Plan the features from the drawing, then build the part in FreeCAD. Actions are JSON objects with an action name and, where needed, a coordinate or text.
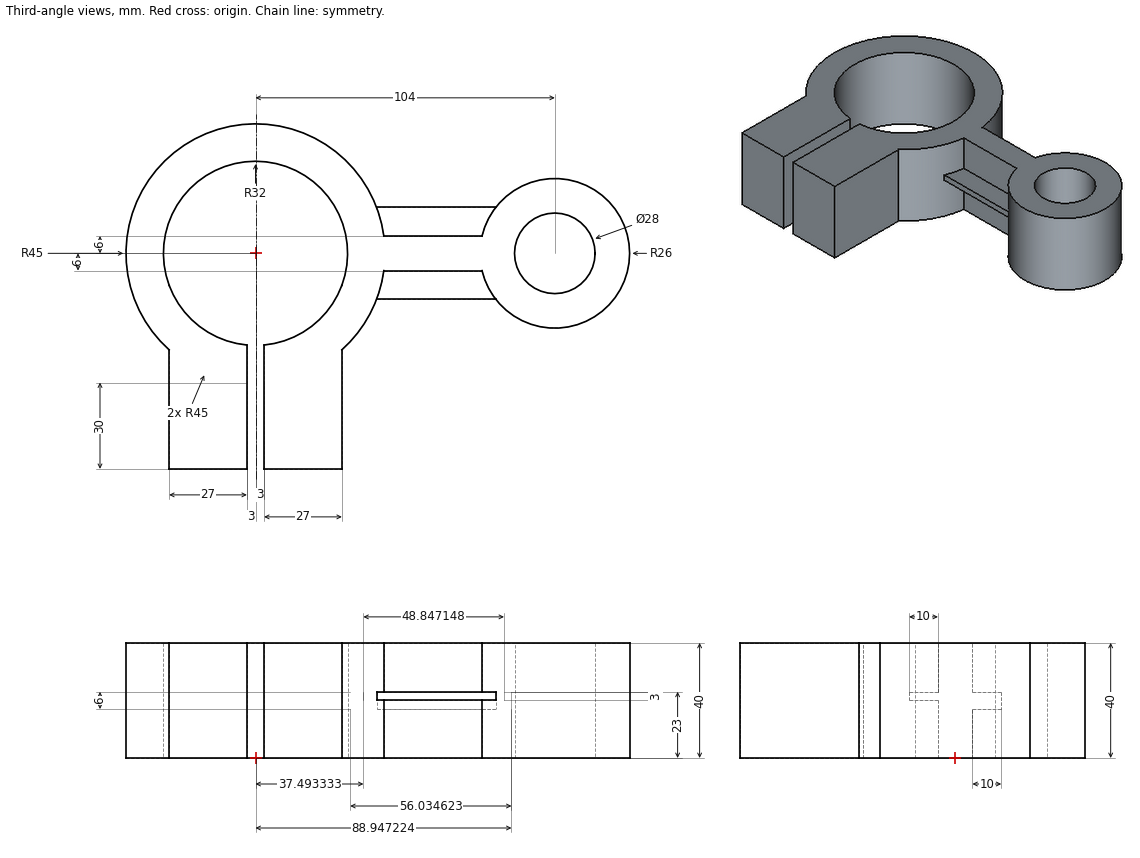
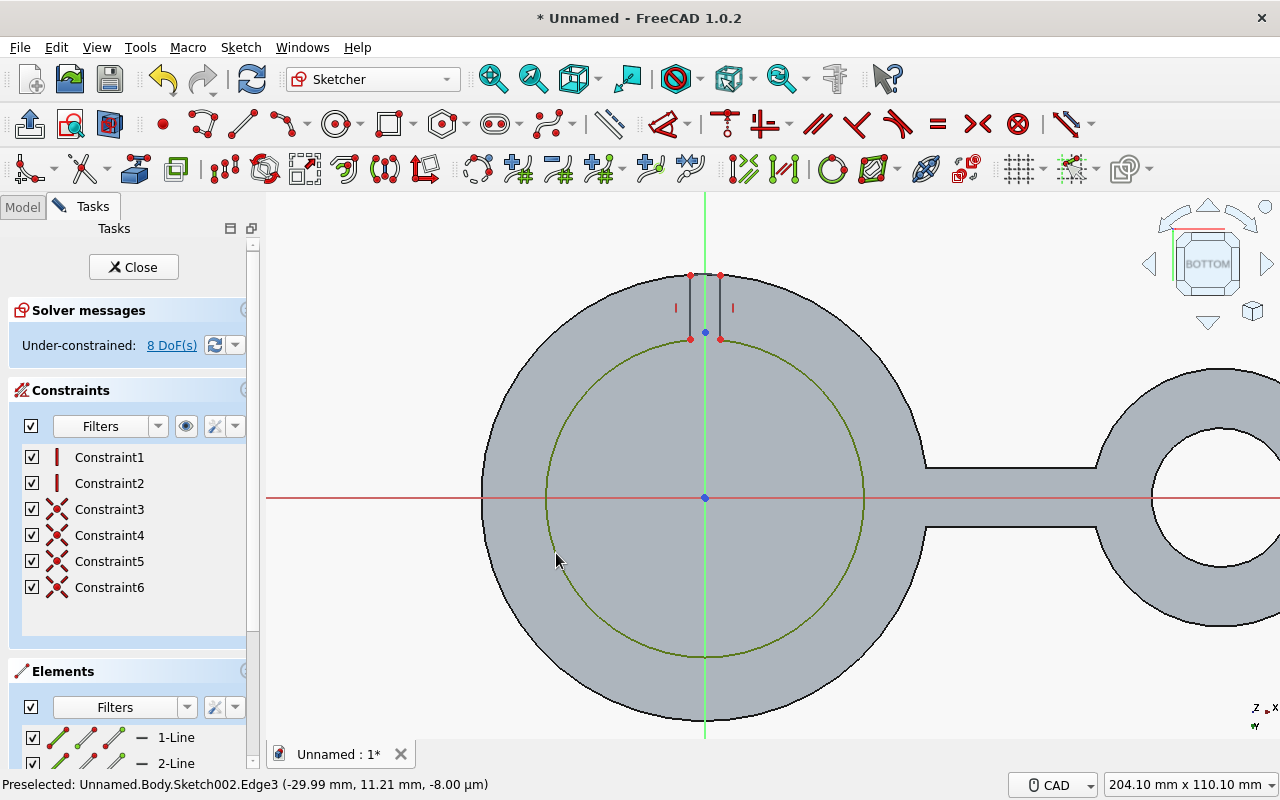
{"action": "left_click", "coordinate": [705, 274]}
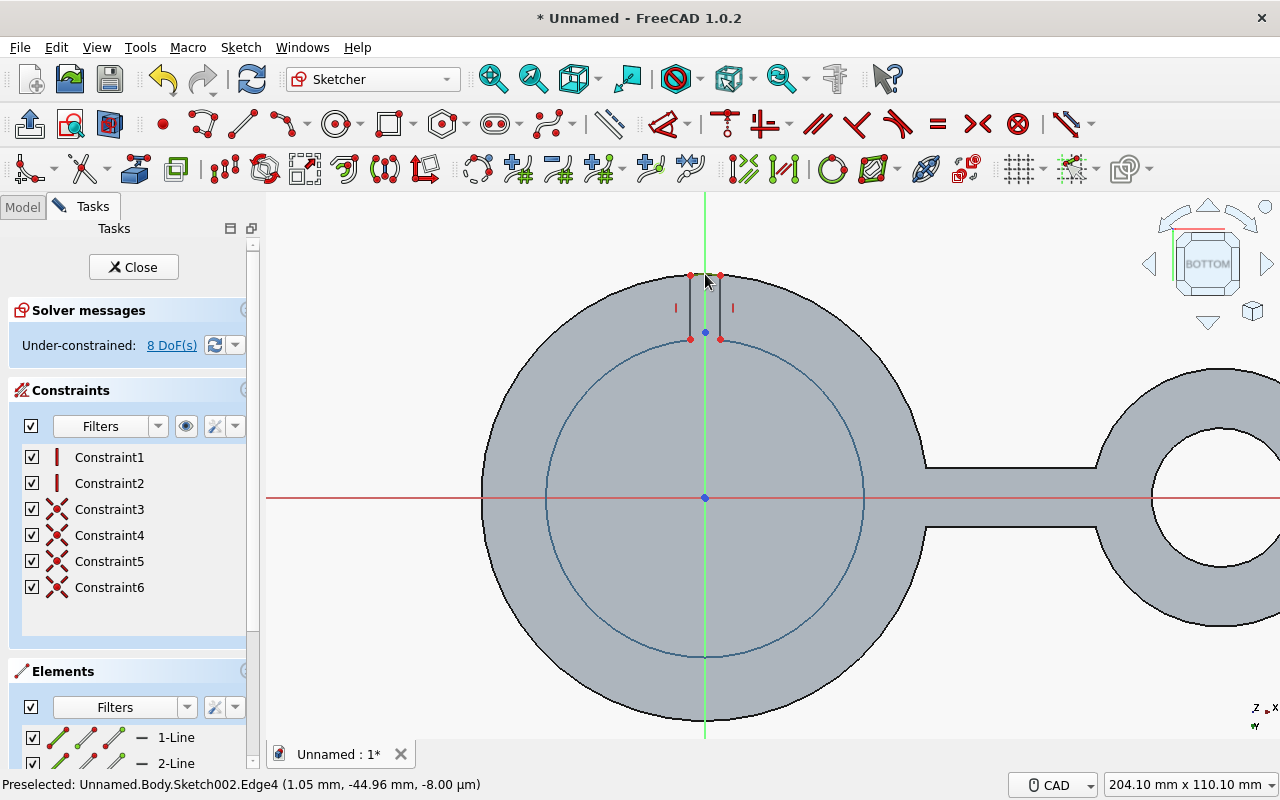
{"action": "key", "text": "c"}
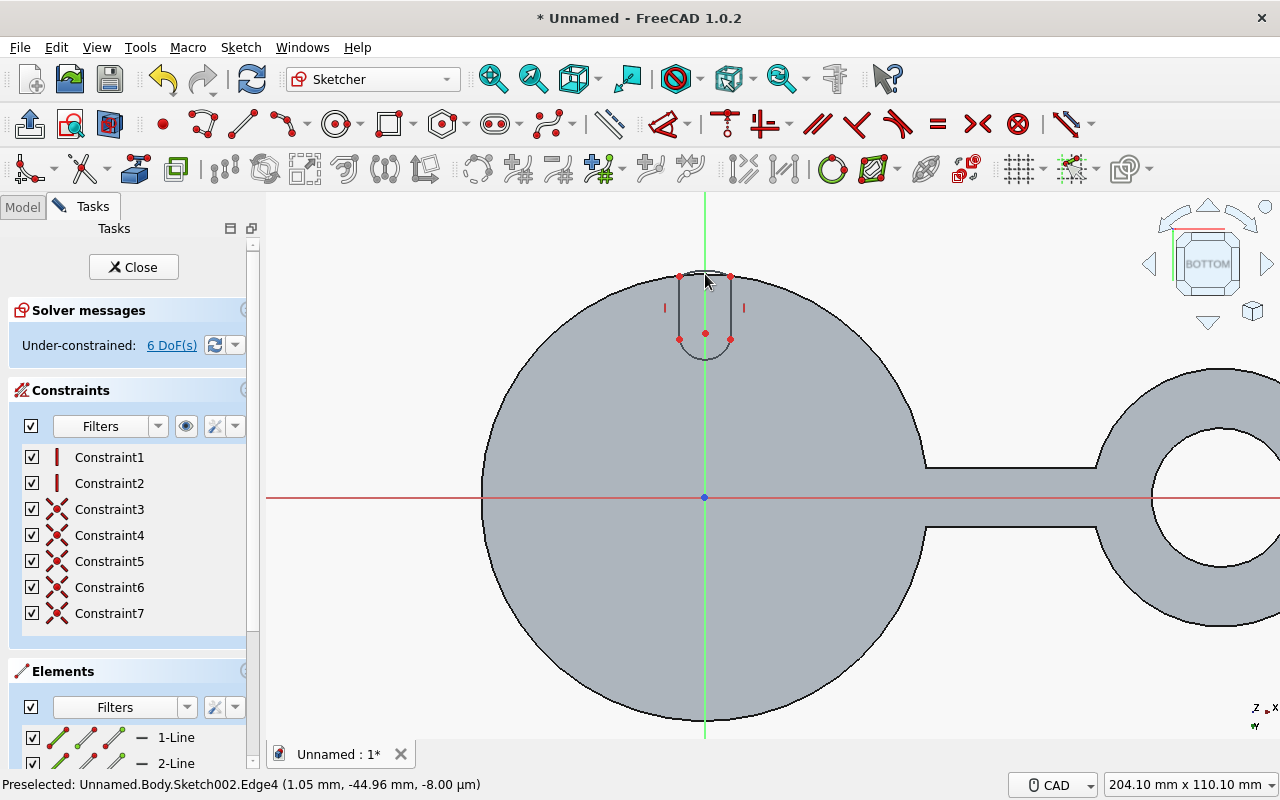
{"action": "scroll", "coordinate": [705, 415], "scroll_direction": "up", "scroll_amount": 3}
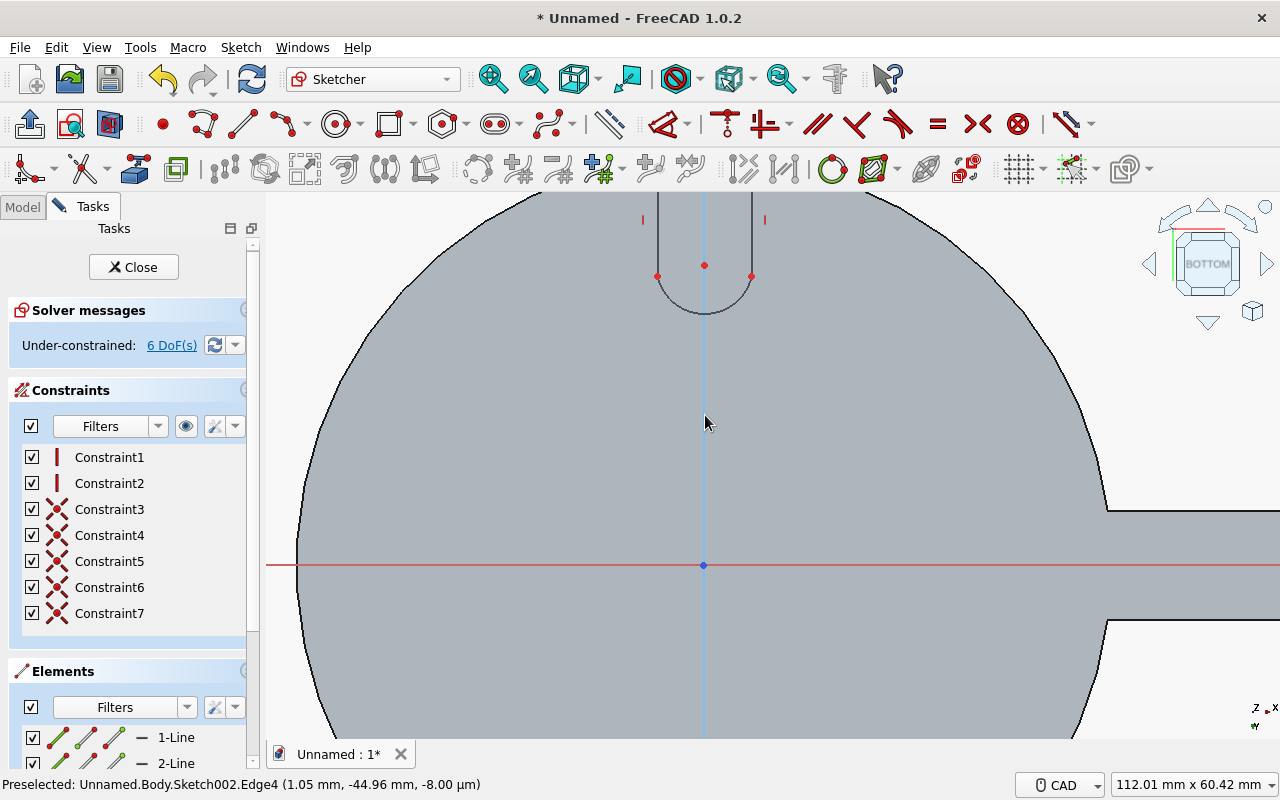
{"action": "left_click_drag", "start_coordinate": [694, 256], "coordinate": [715, 575]}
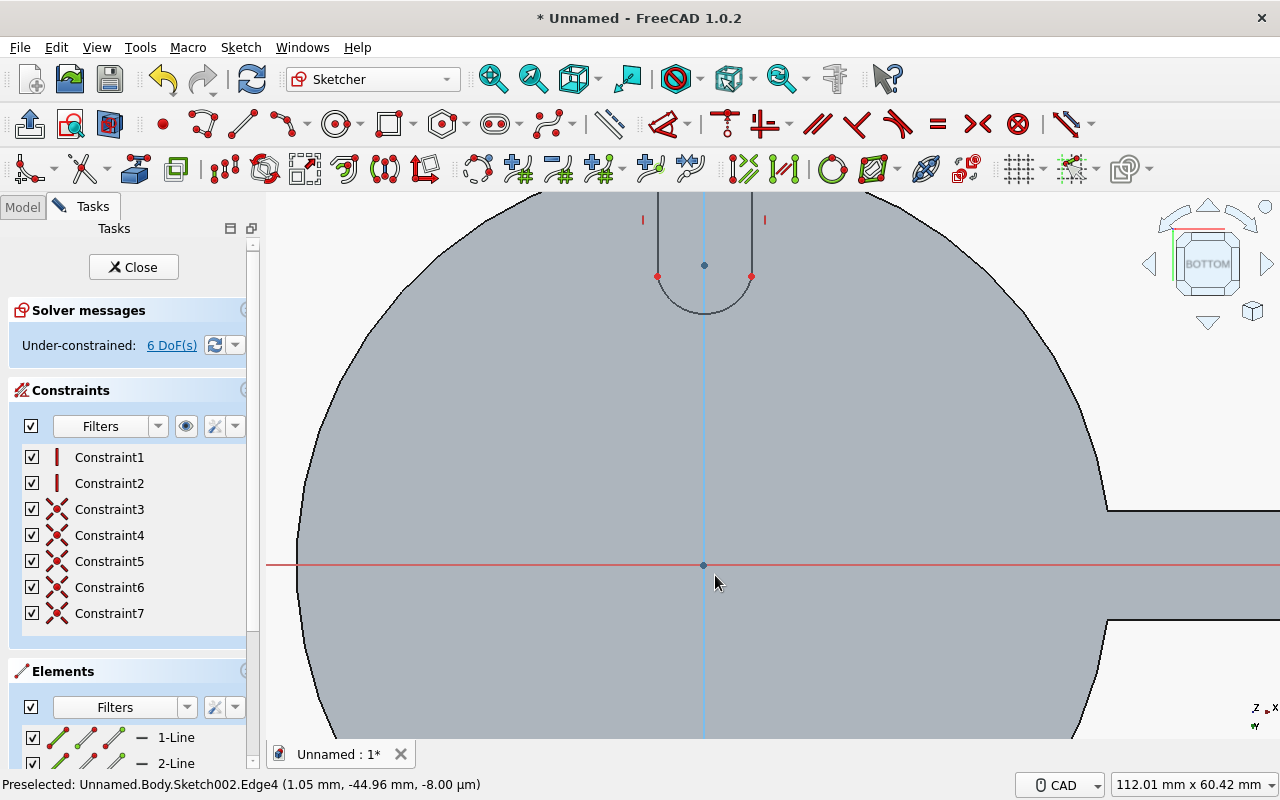
{"action": "left_click", "coordinate": [726, 124]}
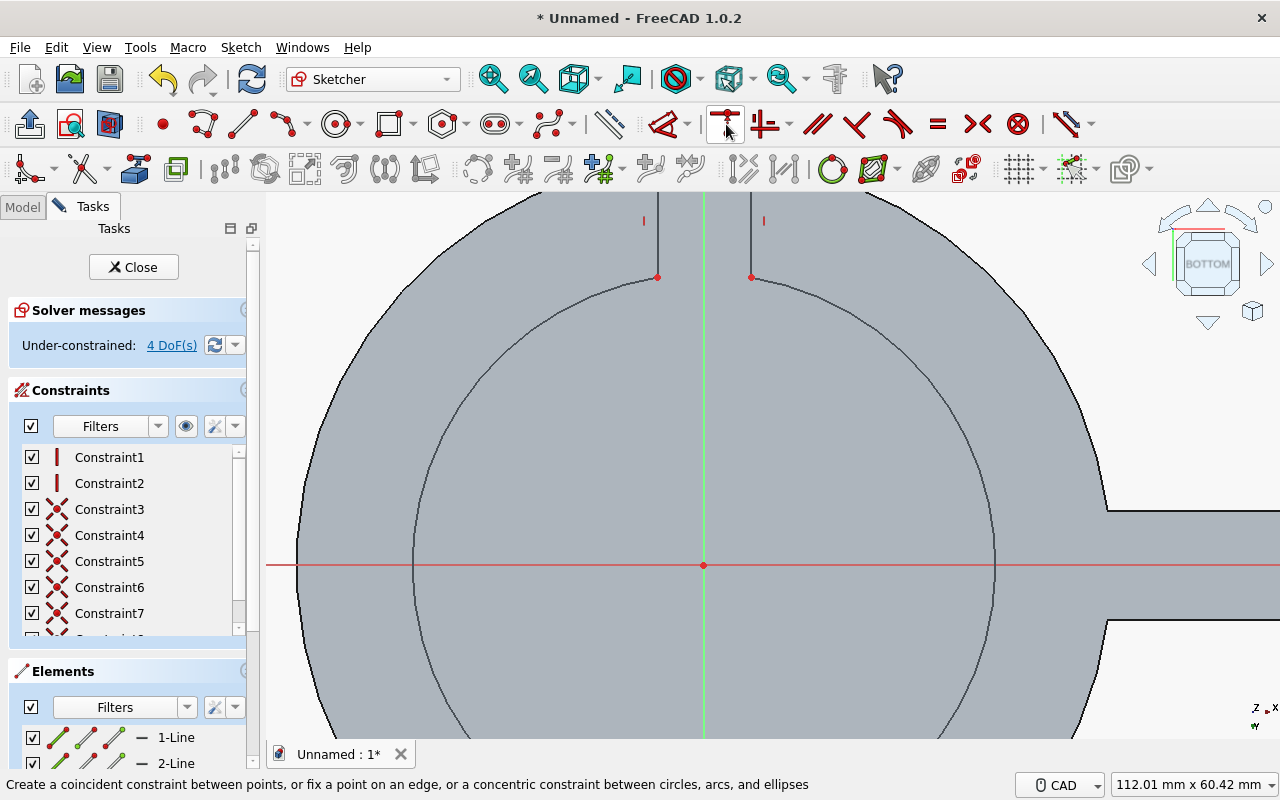
{"action": "key", "text": "d"}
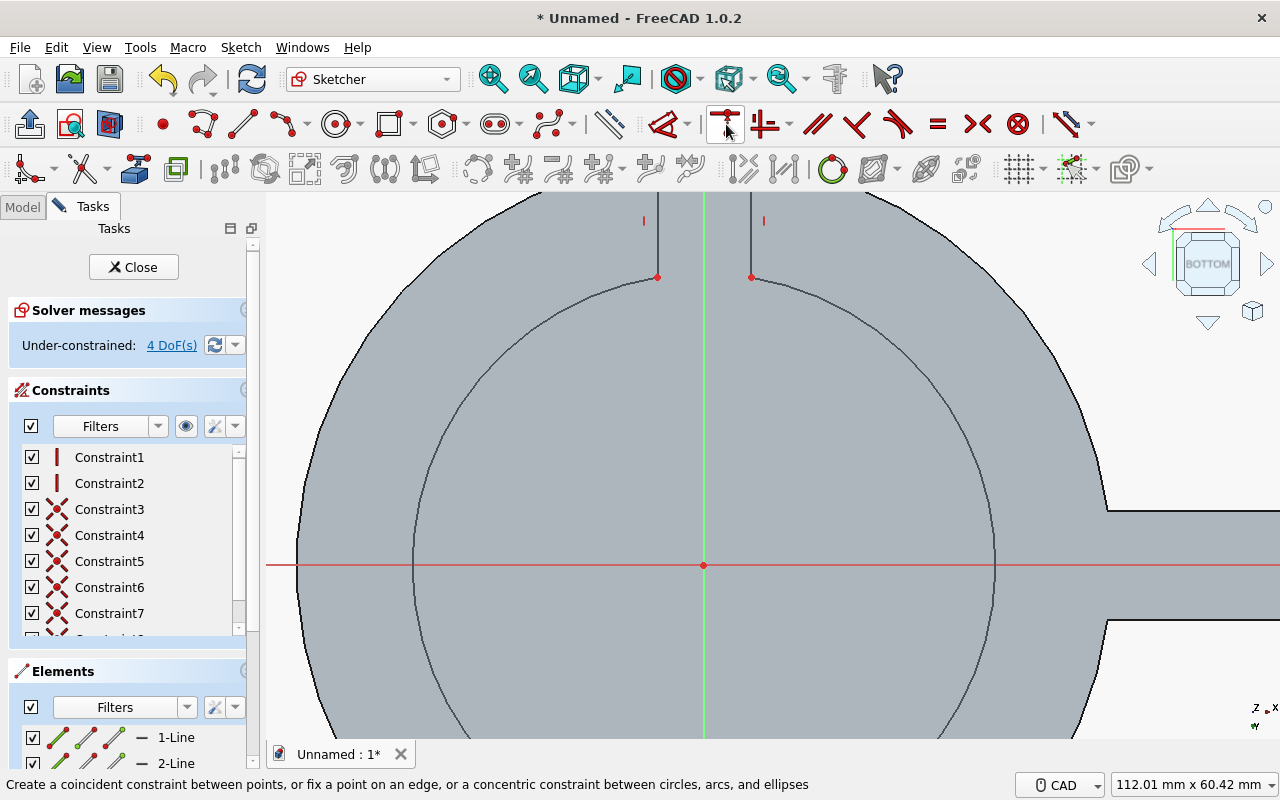
{"action": "left_click", "coordinate": [433, 672]}
{"action": "left_click", "coordinate": [403, 684]}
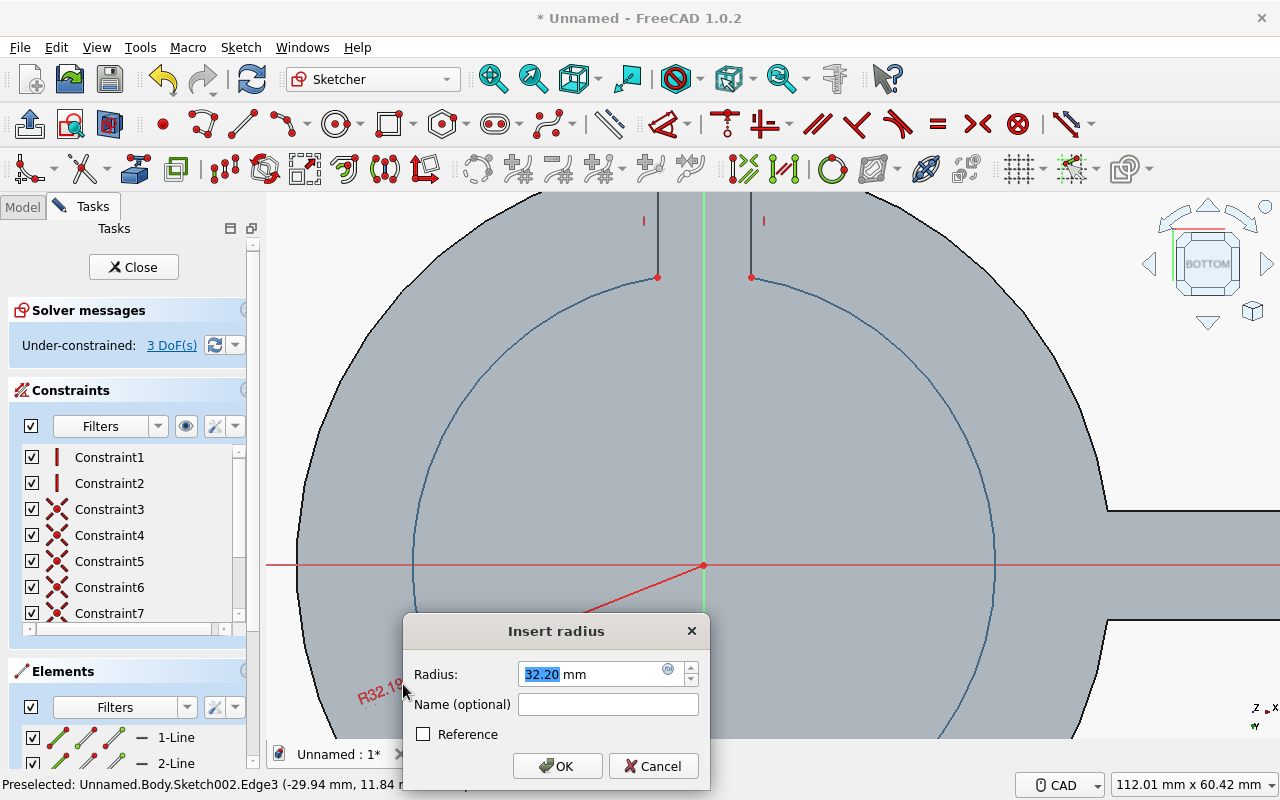
{"action": "type", "text": "32"}
{"action": "key", "text": "Return"}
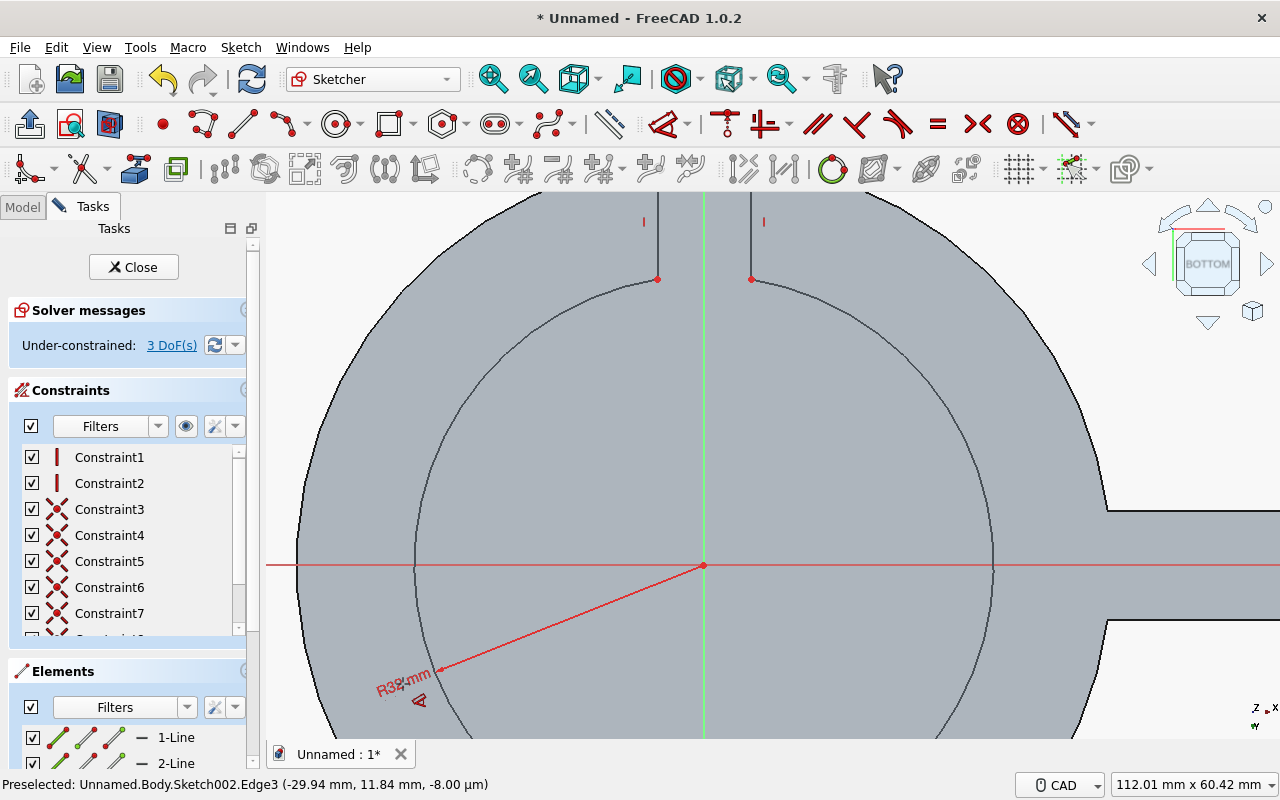
{"action": "scroll", "coordinate": [705, 416], "scroll_direction": "down", "scroll_amount": 3}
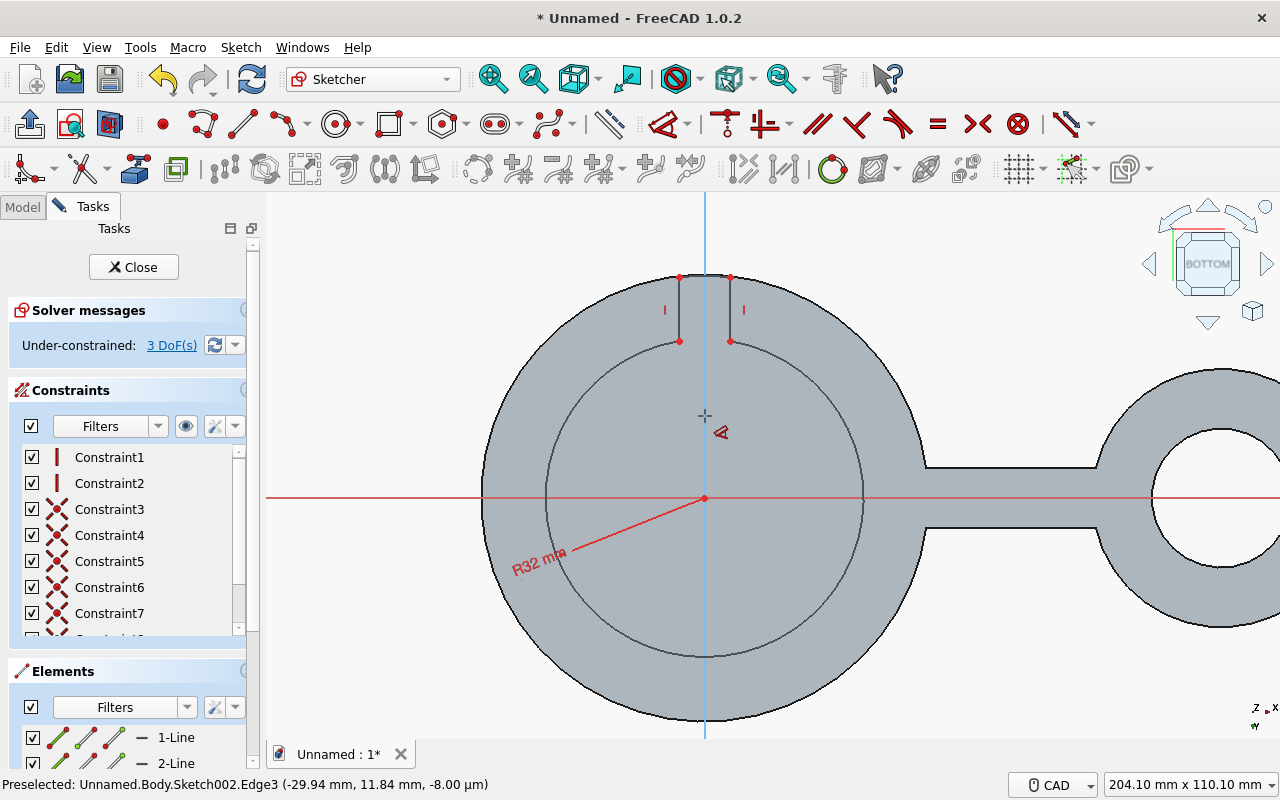
{"action": "scroll", "coordinate": [715, 276], "scroll_direction": "up", "scroll_amount": 2}